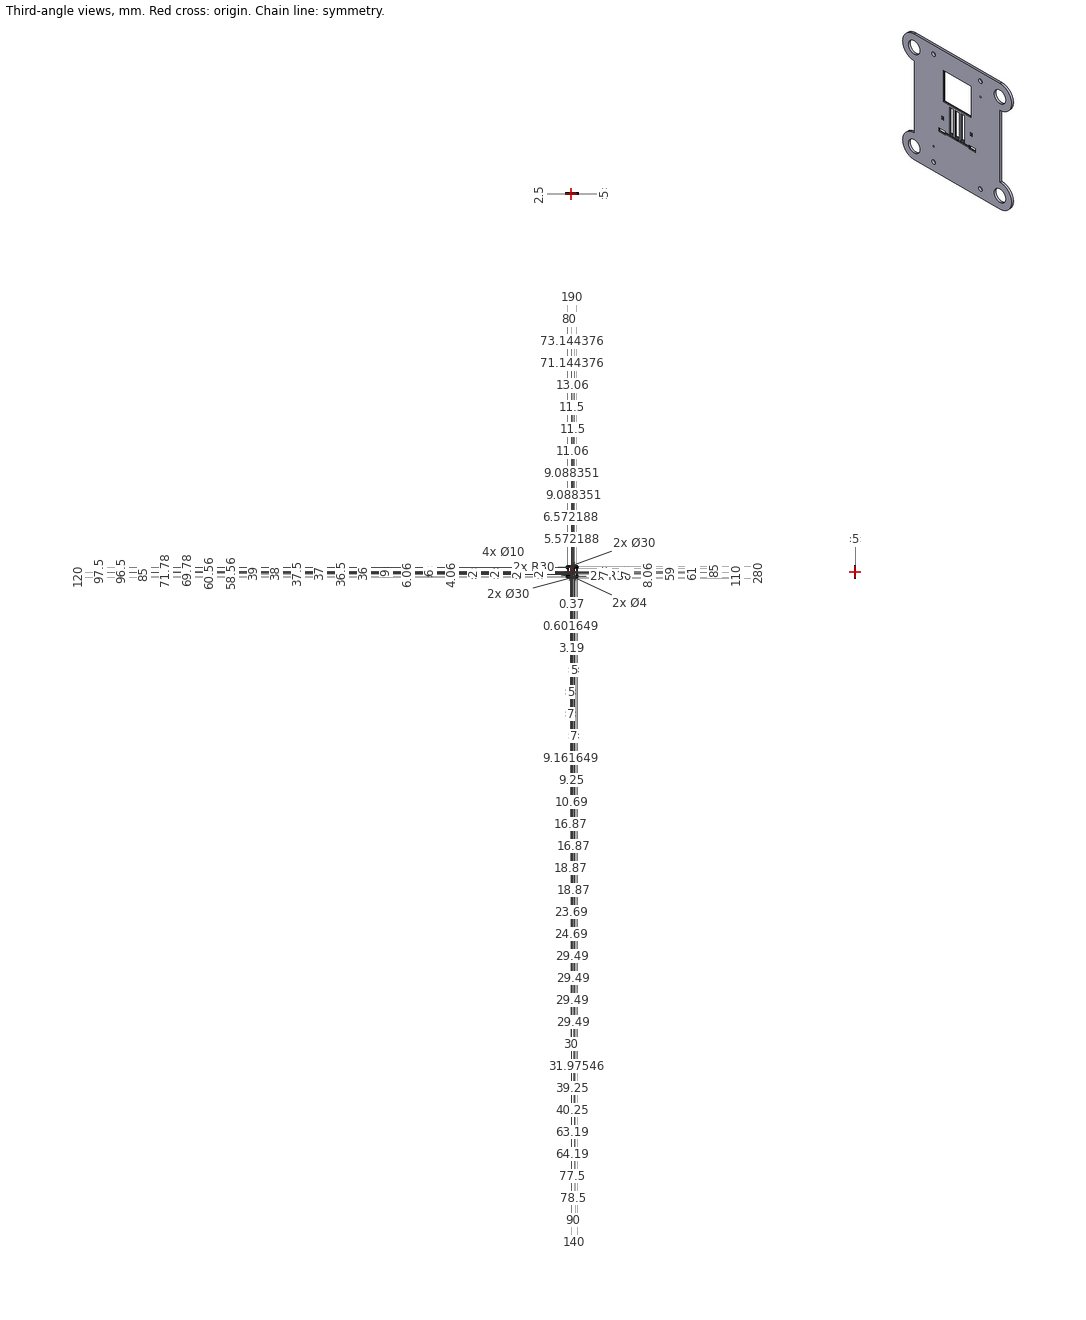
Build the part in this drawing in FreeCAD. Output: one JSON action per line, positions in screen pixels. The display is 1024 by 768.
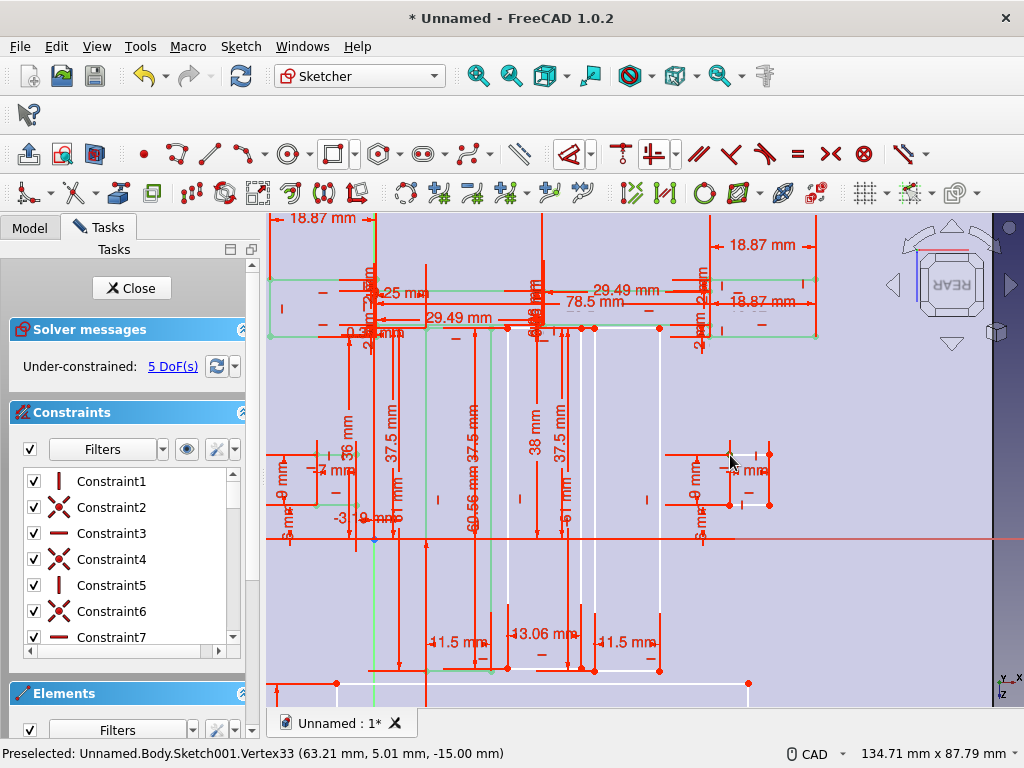
{"action": "left_click", "coordinate": [590, 154]}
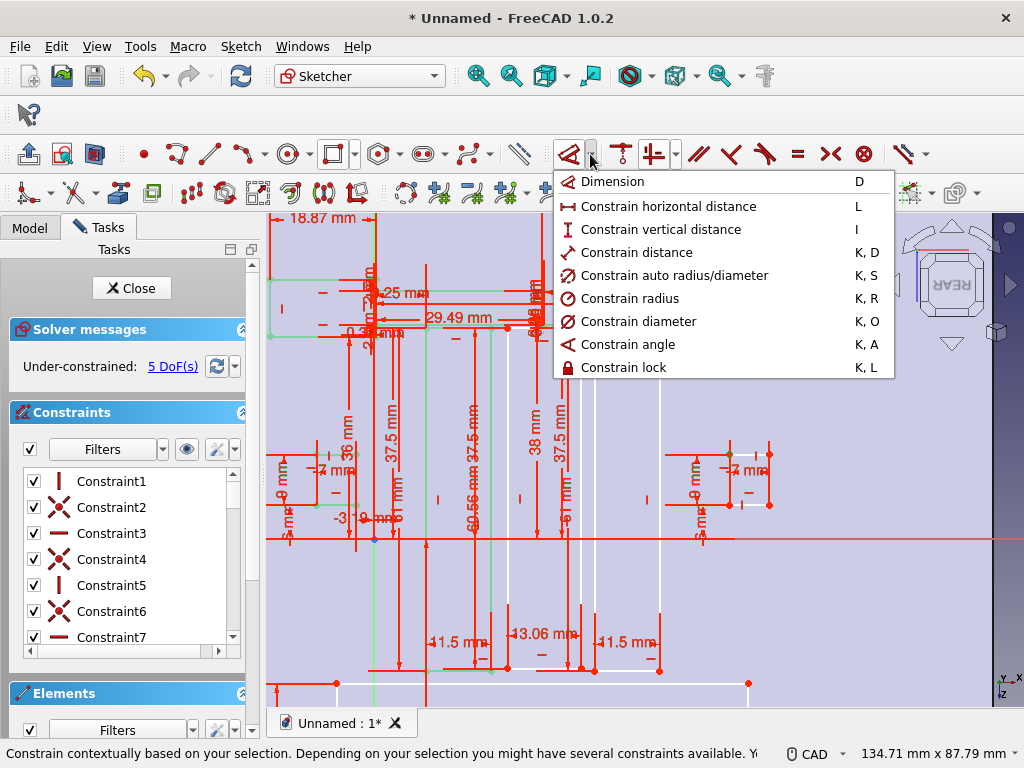
{"action": "left_click", "coordinate": [724, 206]}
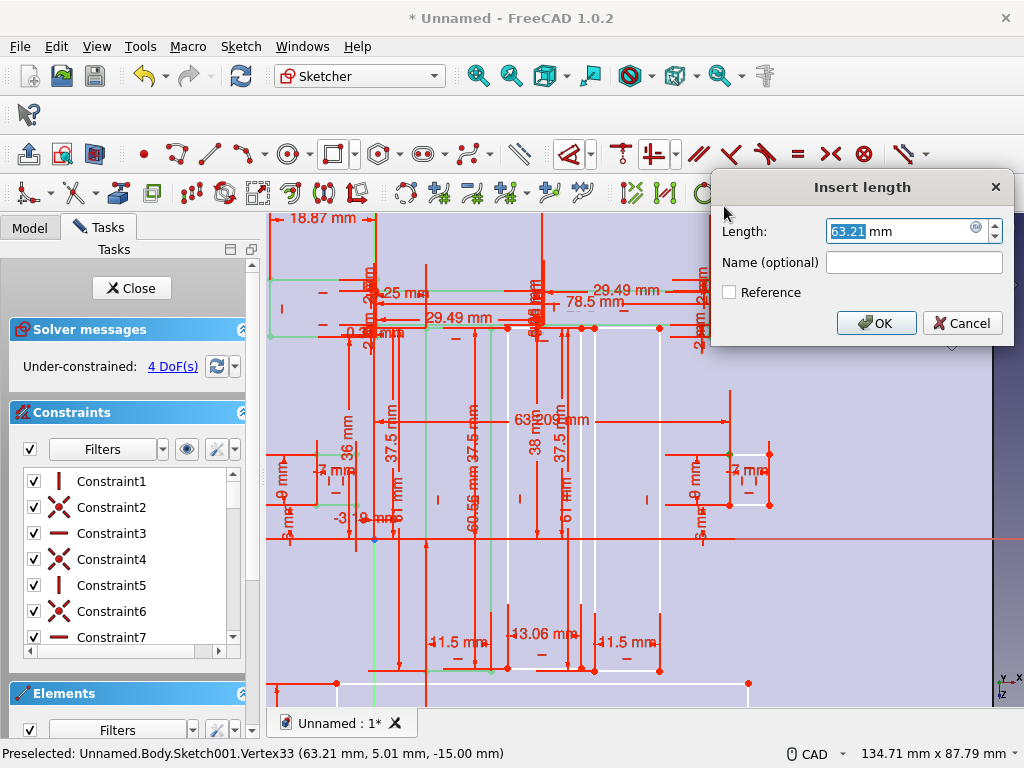
{"action": "type", "text": "63.19"}
{"action": "key", "text": "Return"}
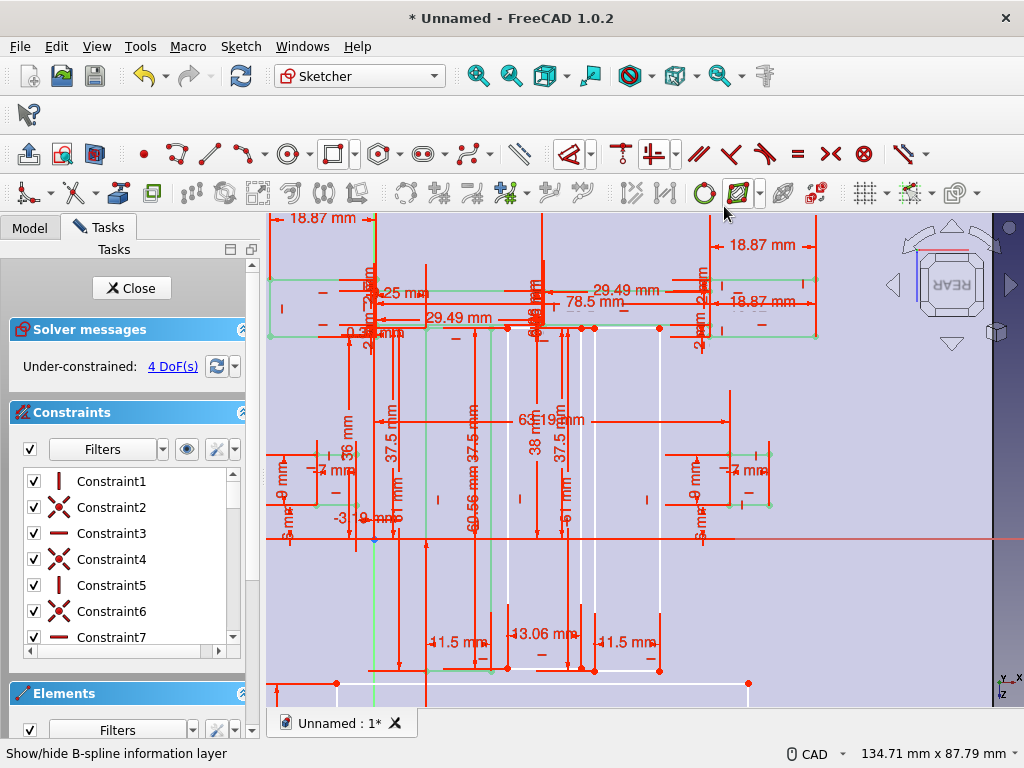
{"action": "left_click", "coordinate": [595, 328]}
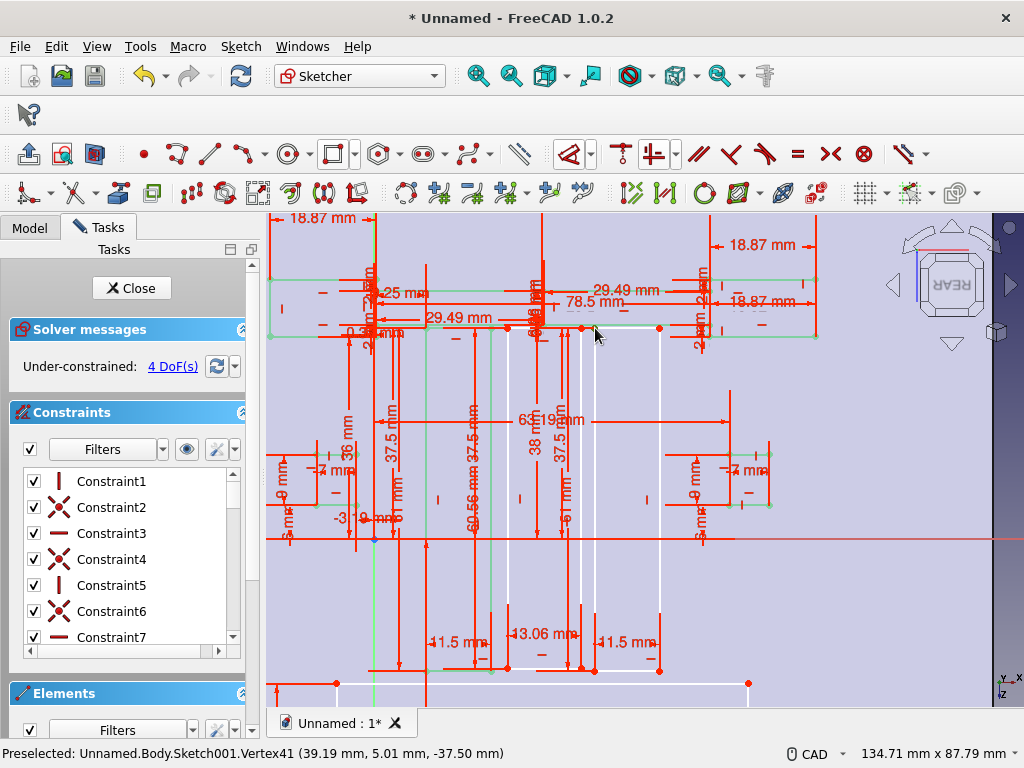
{"action": "key", "text": "l"}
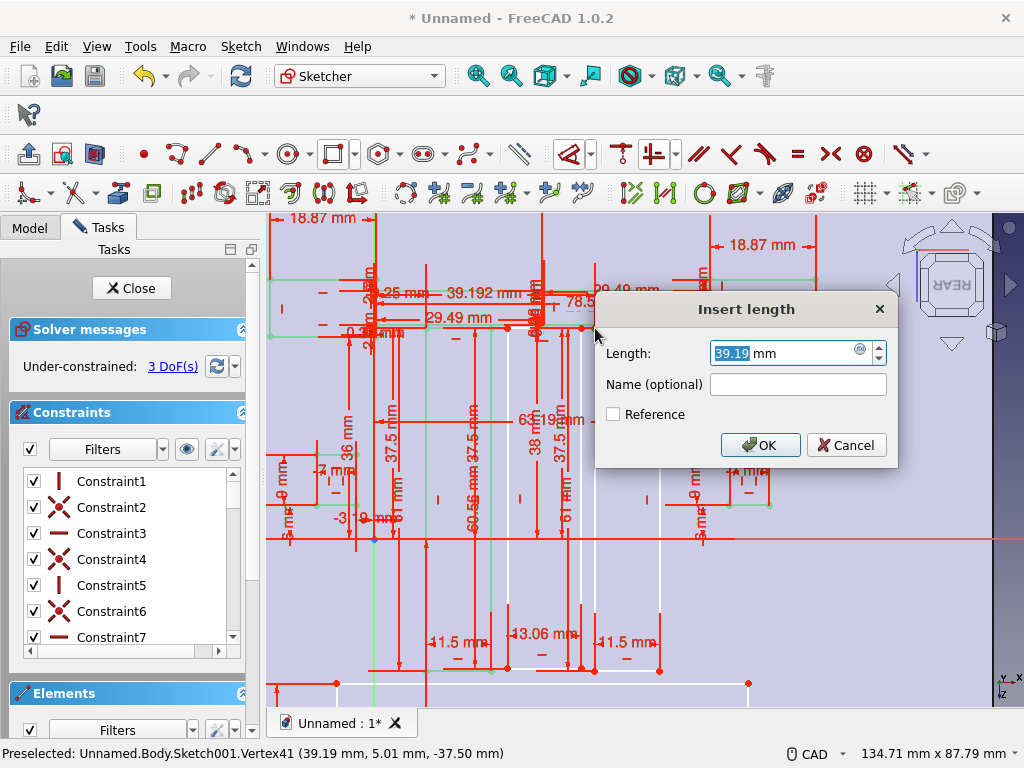
{"action": "type", "text": "39.25"}
{"action": "key", "text": "Return"}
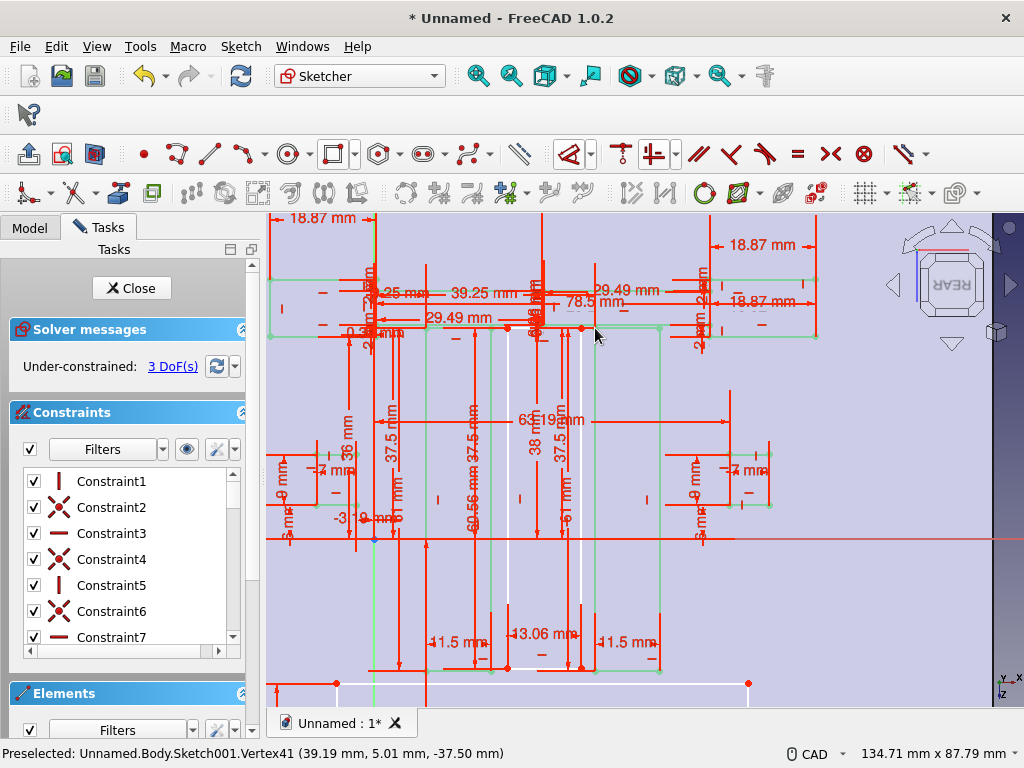
{"action": "left_click", "coordinate": [508, 328]}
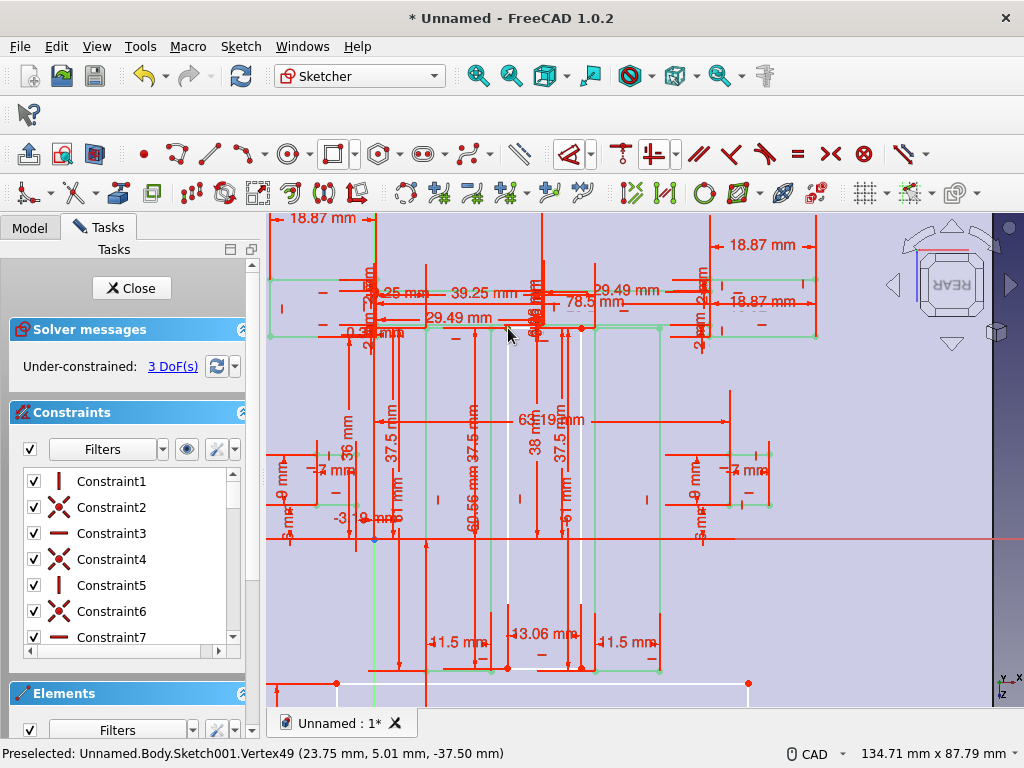
{"action": "key", "text": "l"}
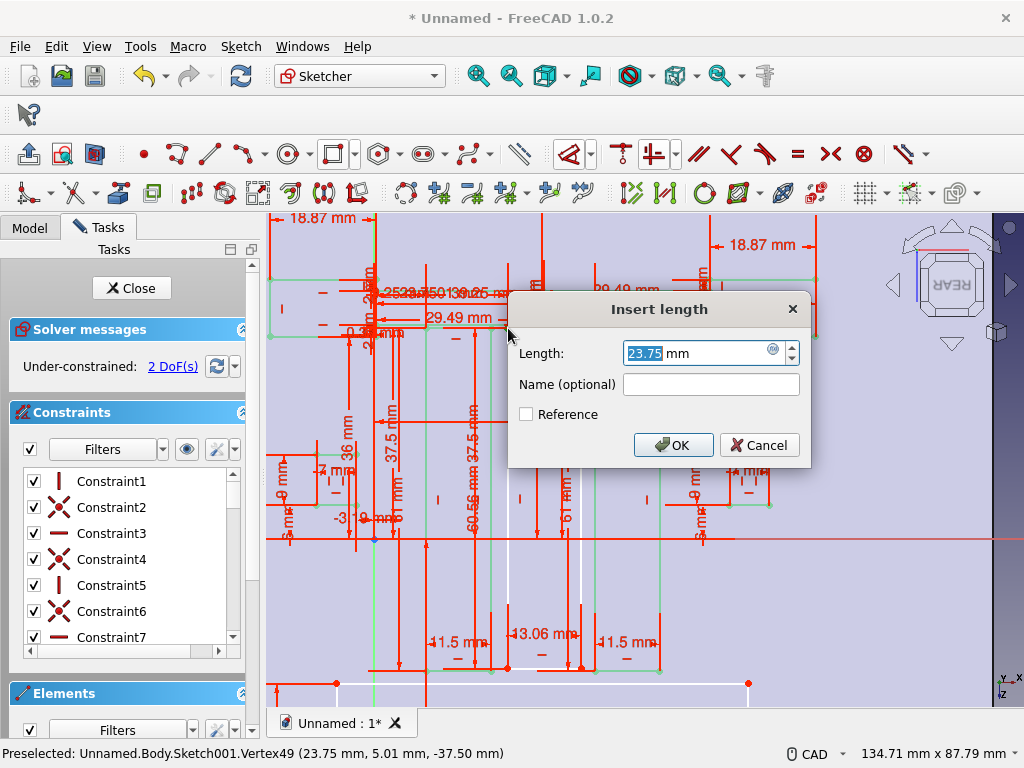
{"action": "type", "text": "23.69"}
{"action": "key", "text": "Return"}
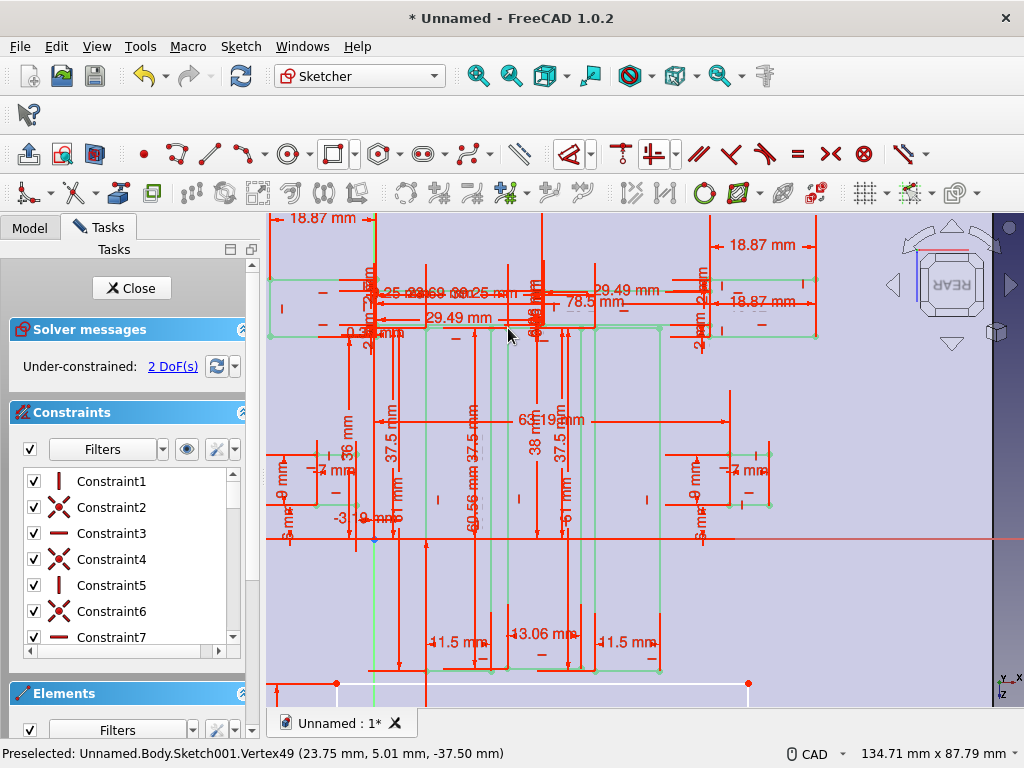
{"action": "scroll", "coordinate": [596, 330], "scroll_direction": "down", "scroll_amount": 5}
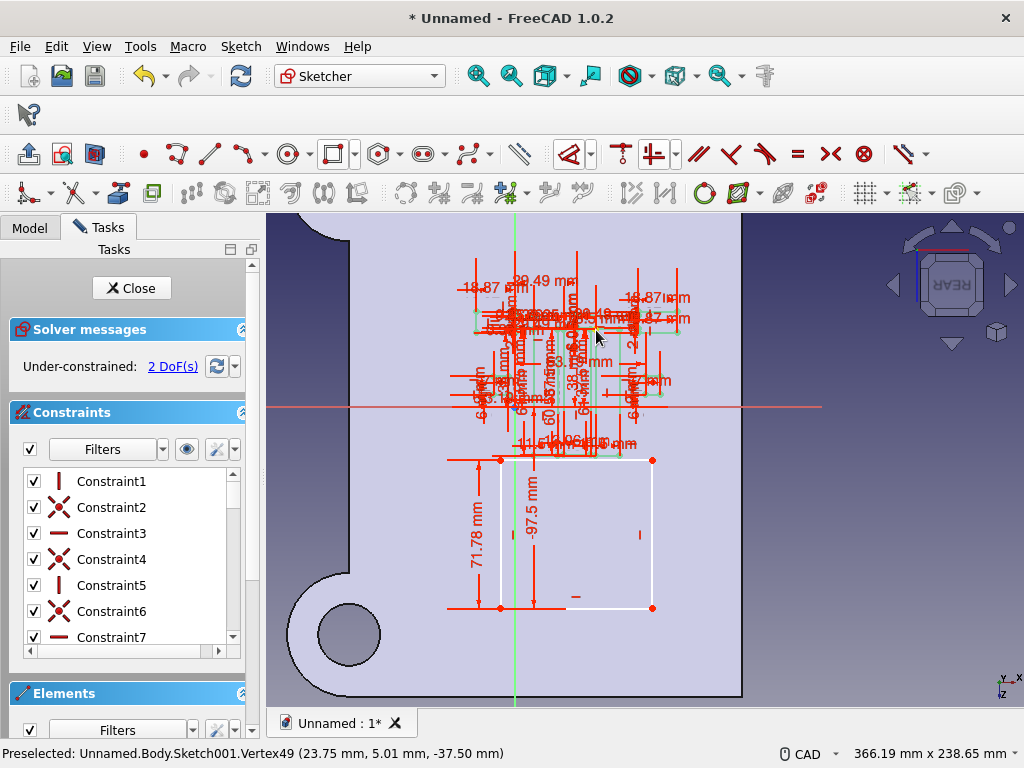
{"action": "left_click", "coordinate": [546, 609]}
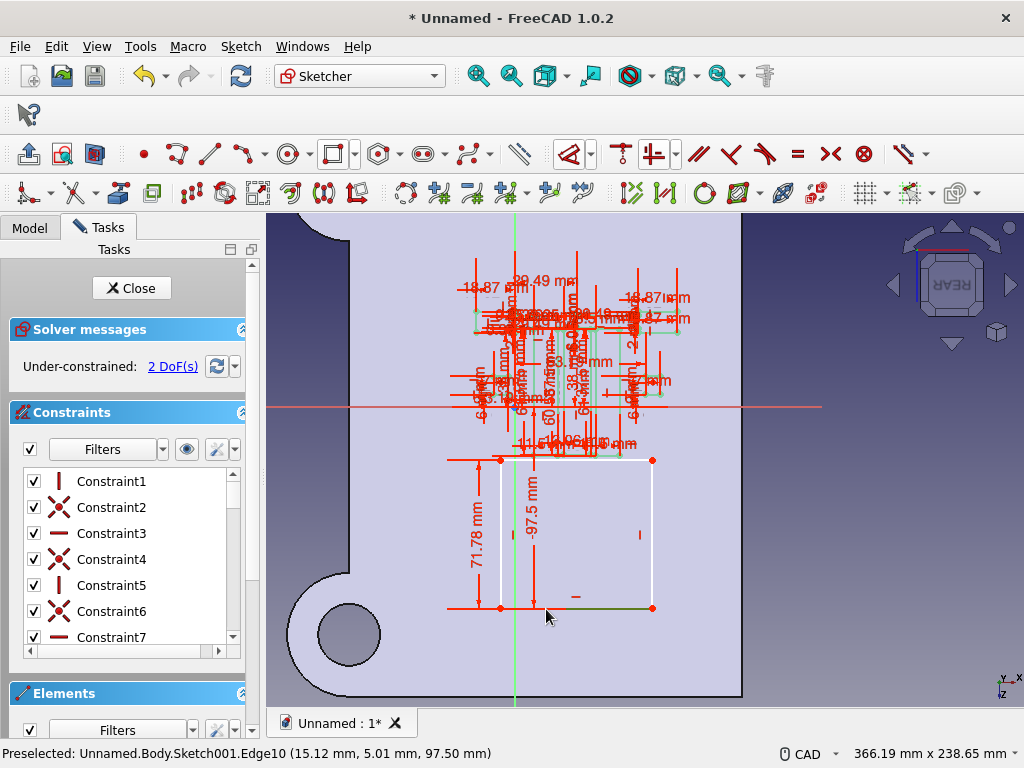
{"action": "key", "text": "l"}